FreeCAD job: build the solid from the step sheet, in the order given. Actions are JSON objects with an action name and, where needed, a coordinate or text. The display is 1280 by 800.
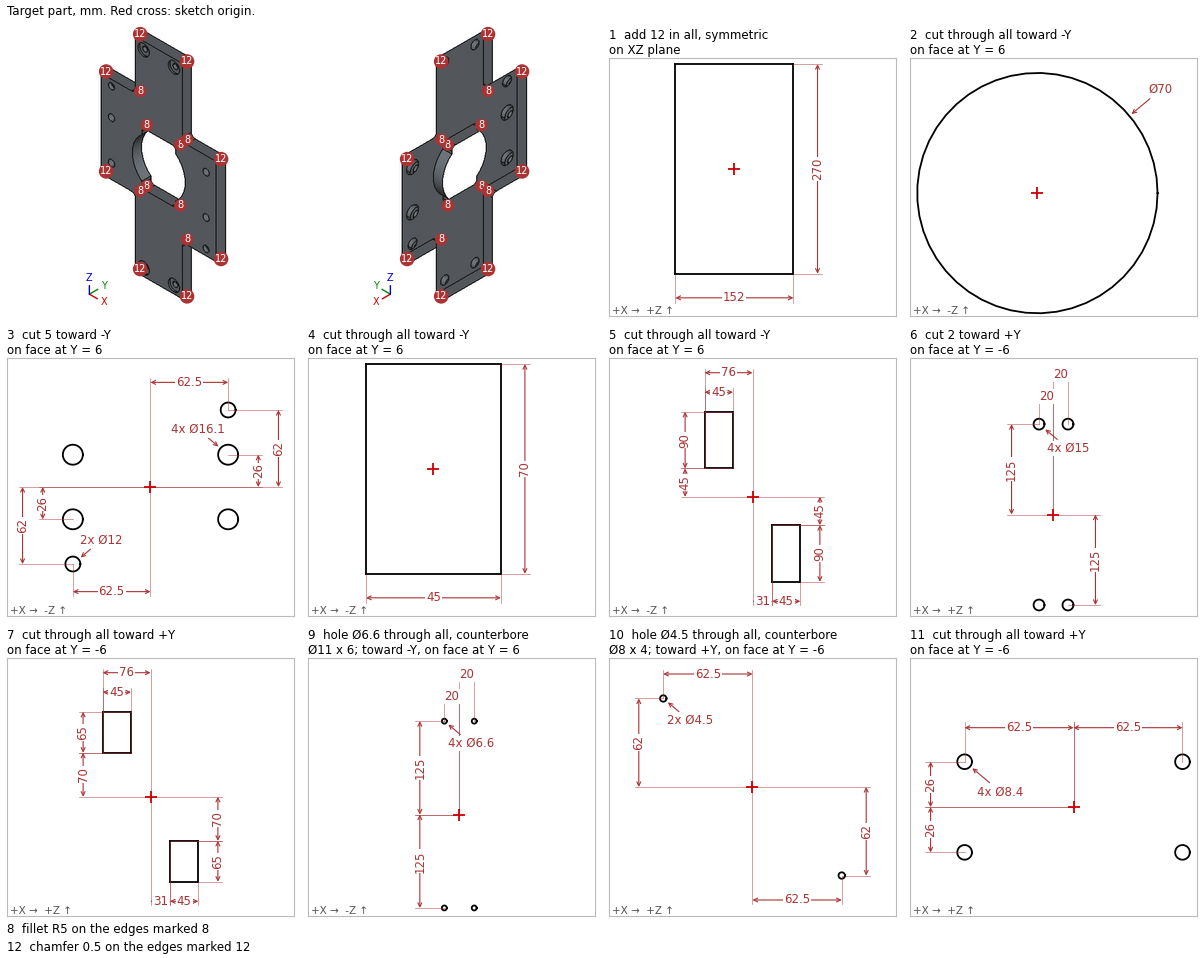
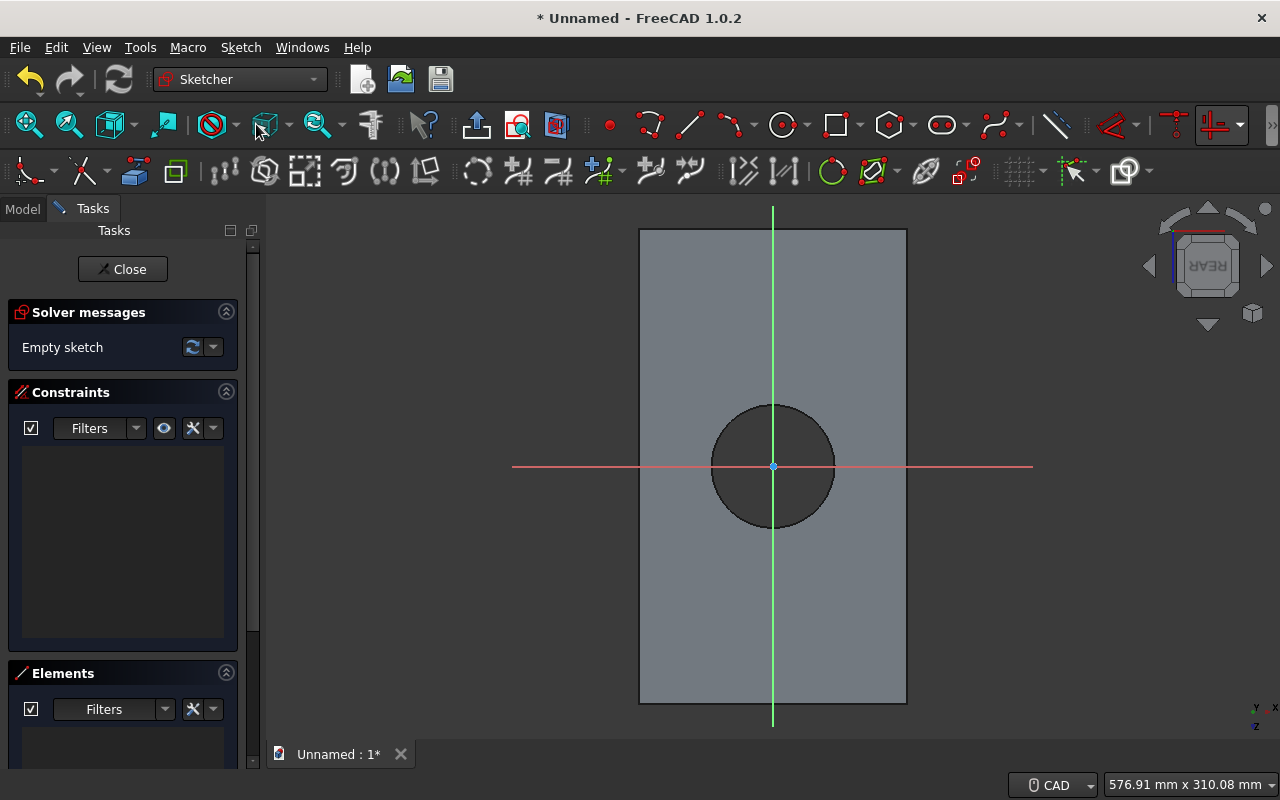
{"action": "scroll", "coordinate": [912, 466], "scroll_direction": "up", "scroll_amount": 2}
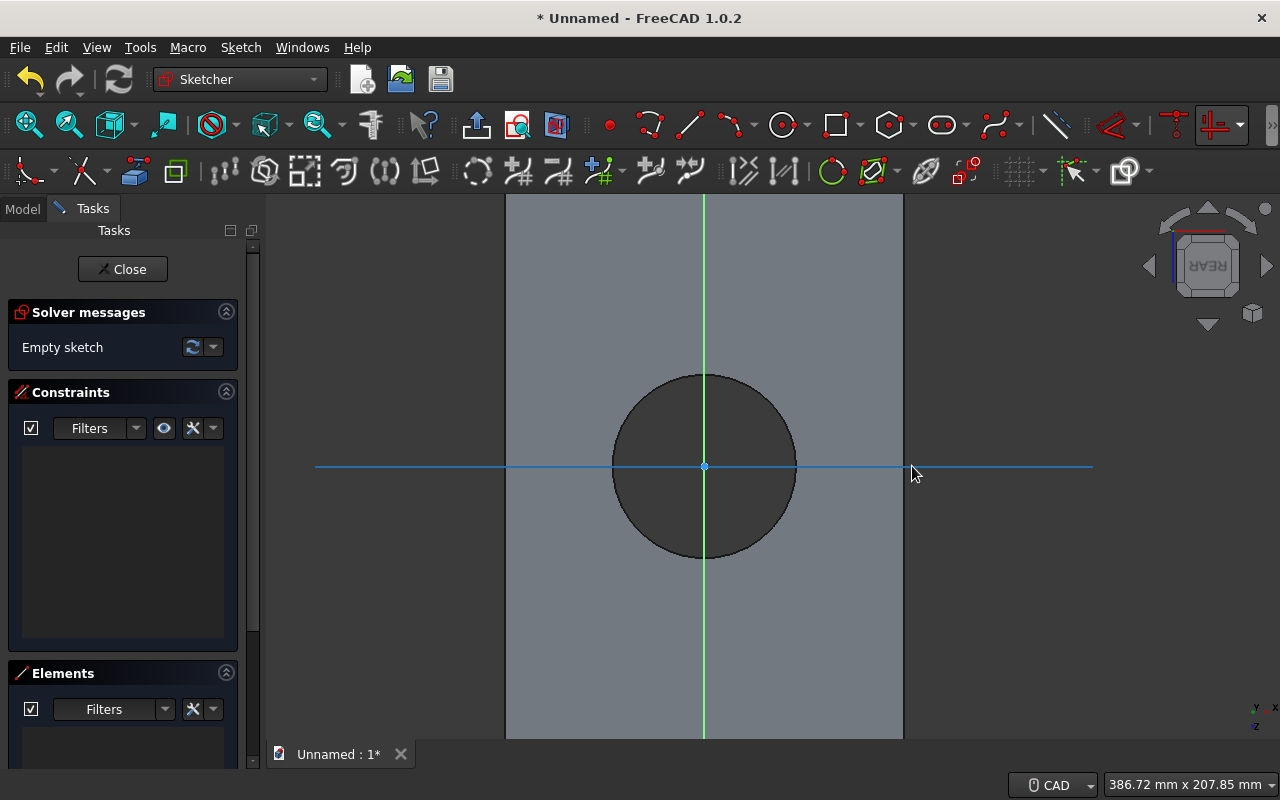
{"action": "left_click", "coordinate": [784, 126]}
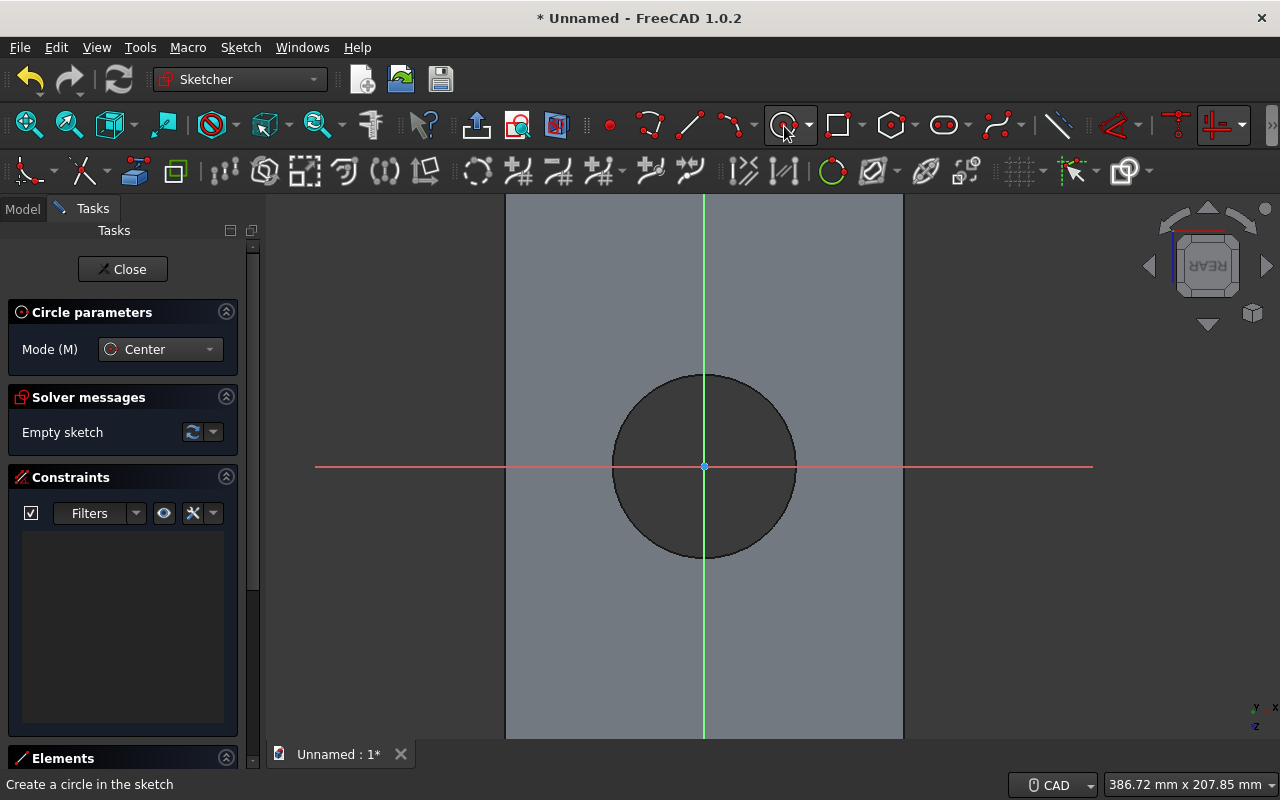
{"action": "scroll", "coordinate": [868, 304], "scroll_direction": "up", "scroll_amount": 2}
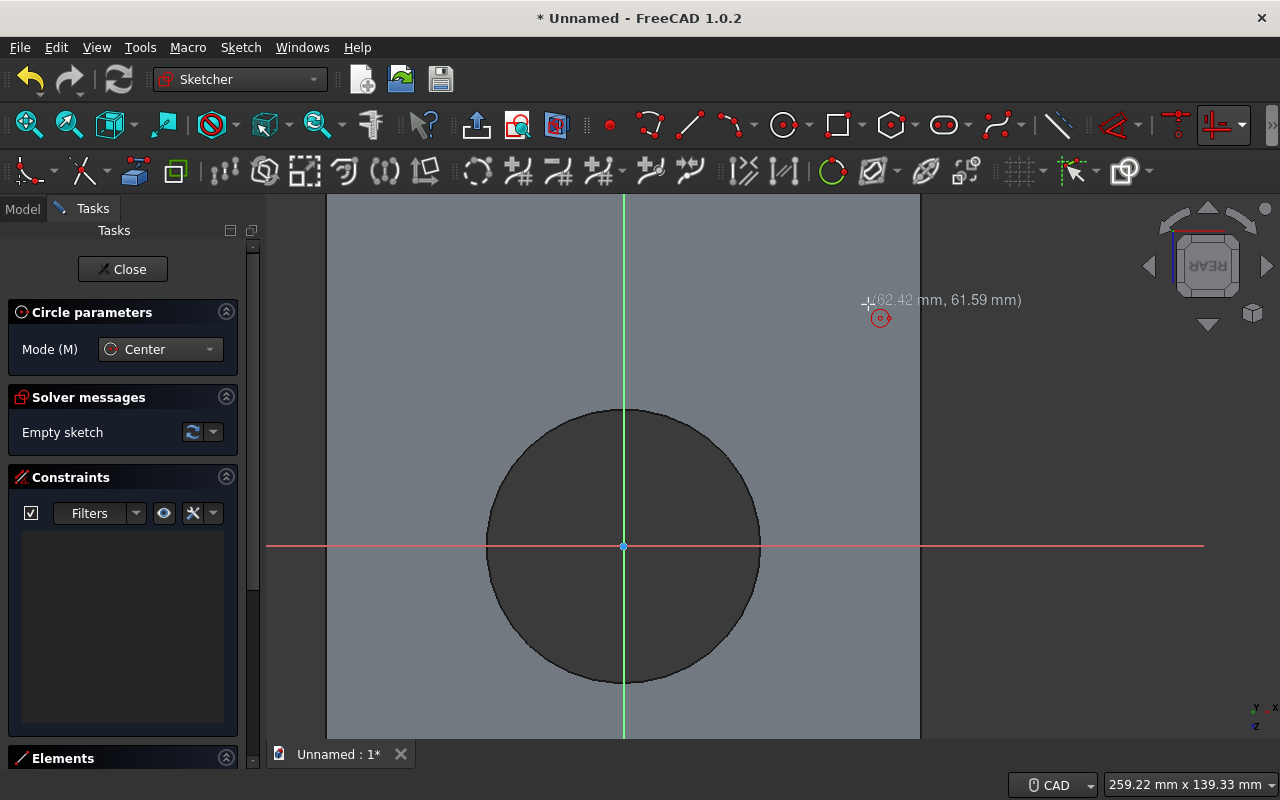
{"action": "left_click", "coordinate": [868, 304]}
{"action": "mouse_move", "coordinate": [885, 287]}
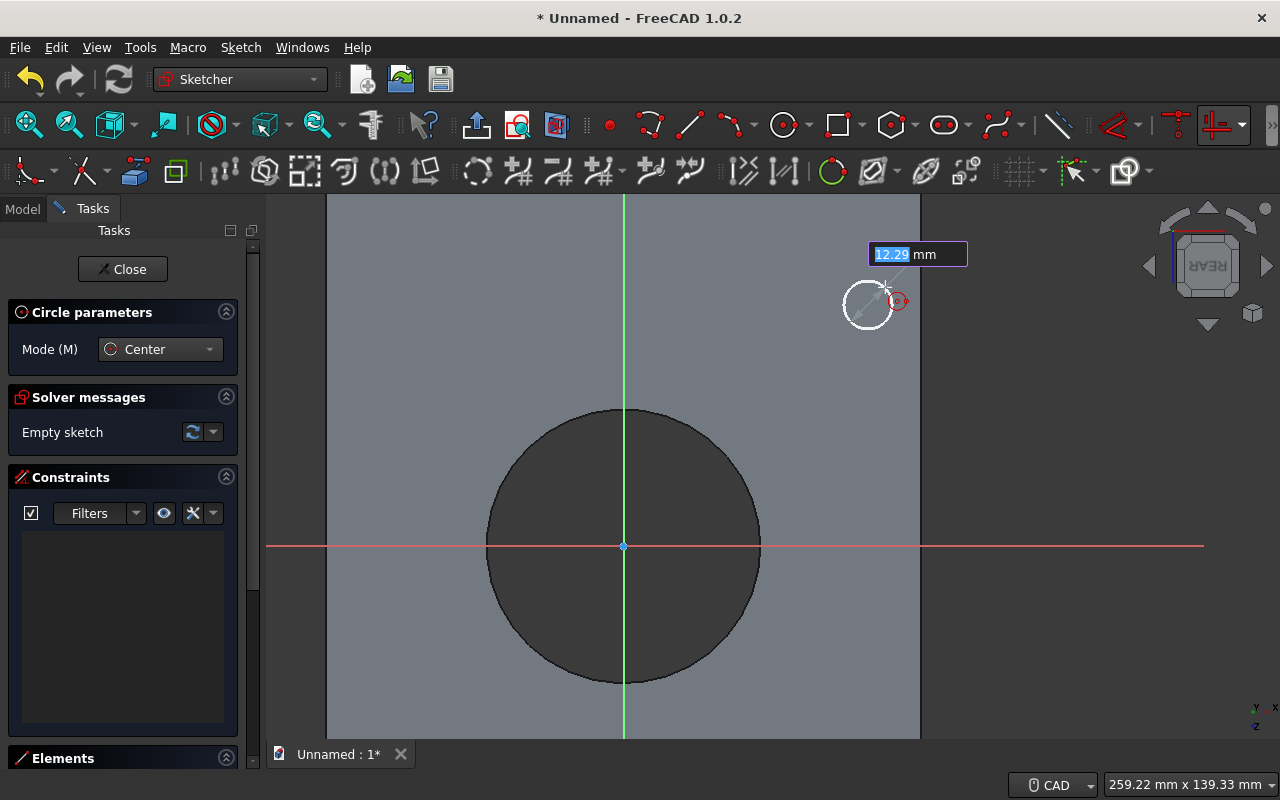
{"action": "type", "text": "12"}
{"action": "key", "text": "Return"}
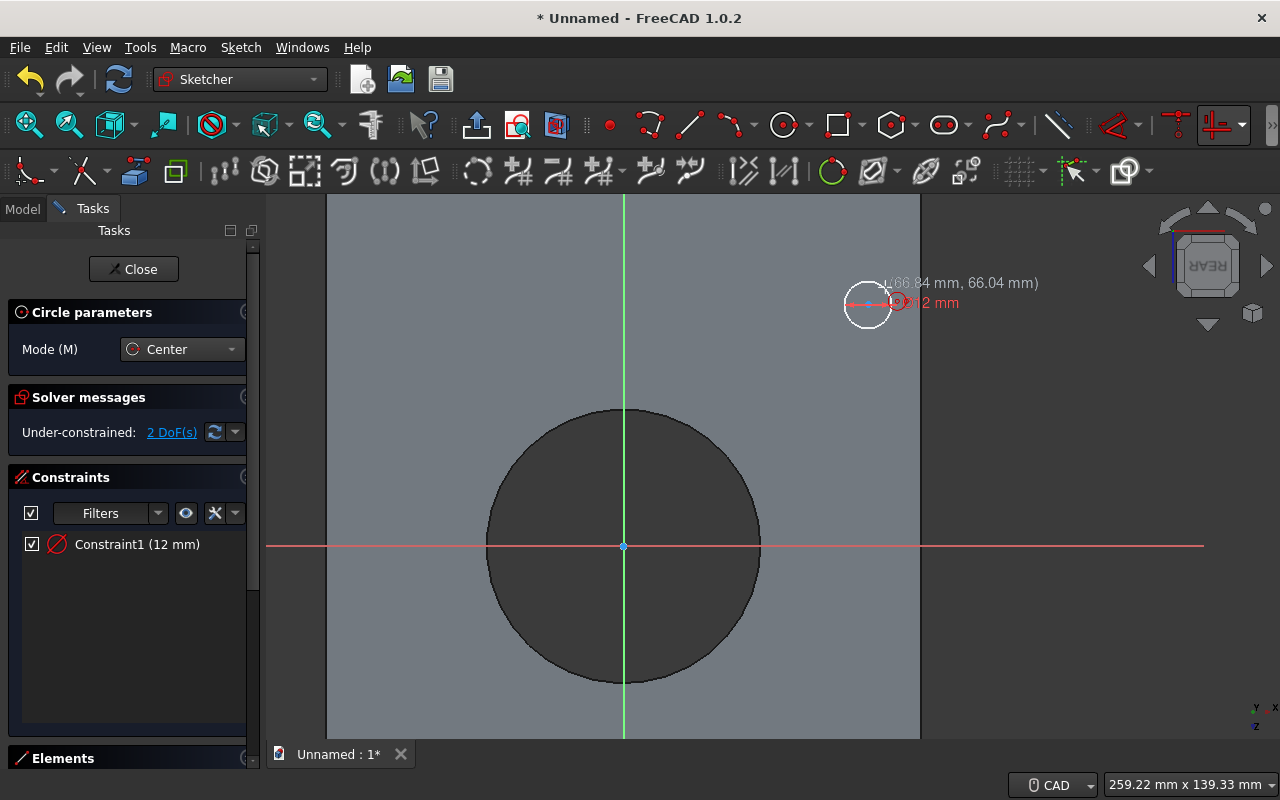
{"action": "scroll", "coordinate": [869, 304], "scroll_direction": "down", "scroll_amount": 2}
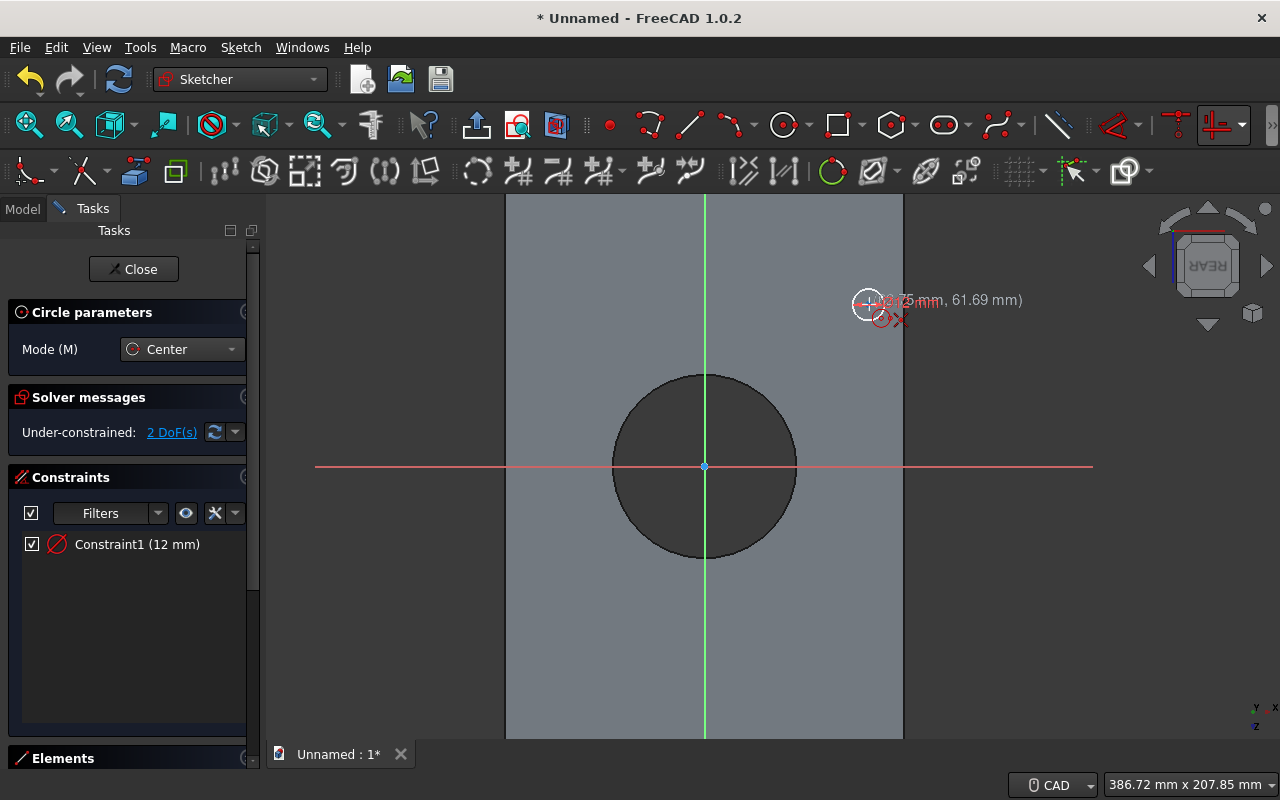
{"action": "scroll", "coordinate": [541, 629], "scroll_direction": "up", "scroll_amount": 2}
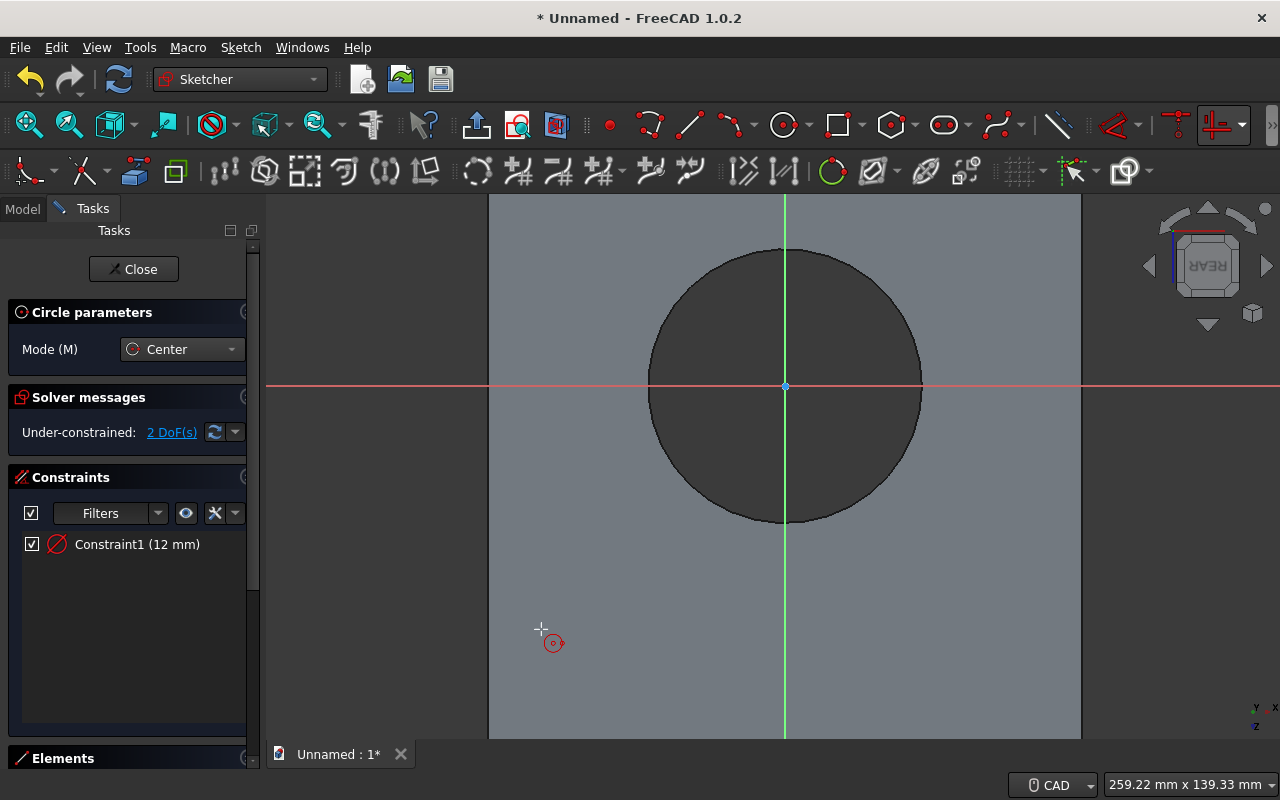
{"action": "left_click", "coordinate": [541, 629]}
{"action": "mouse_move", "coordinate": [557, 612]}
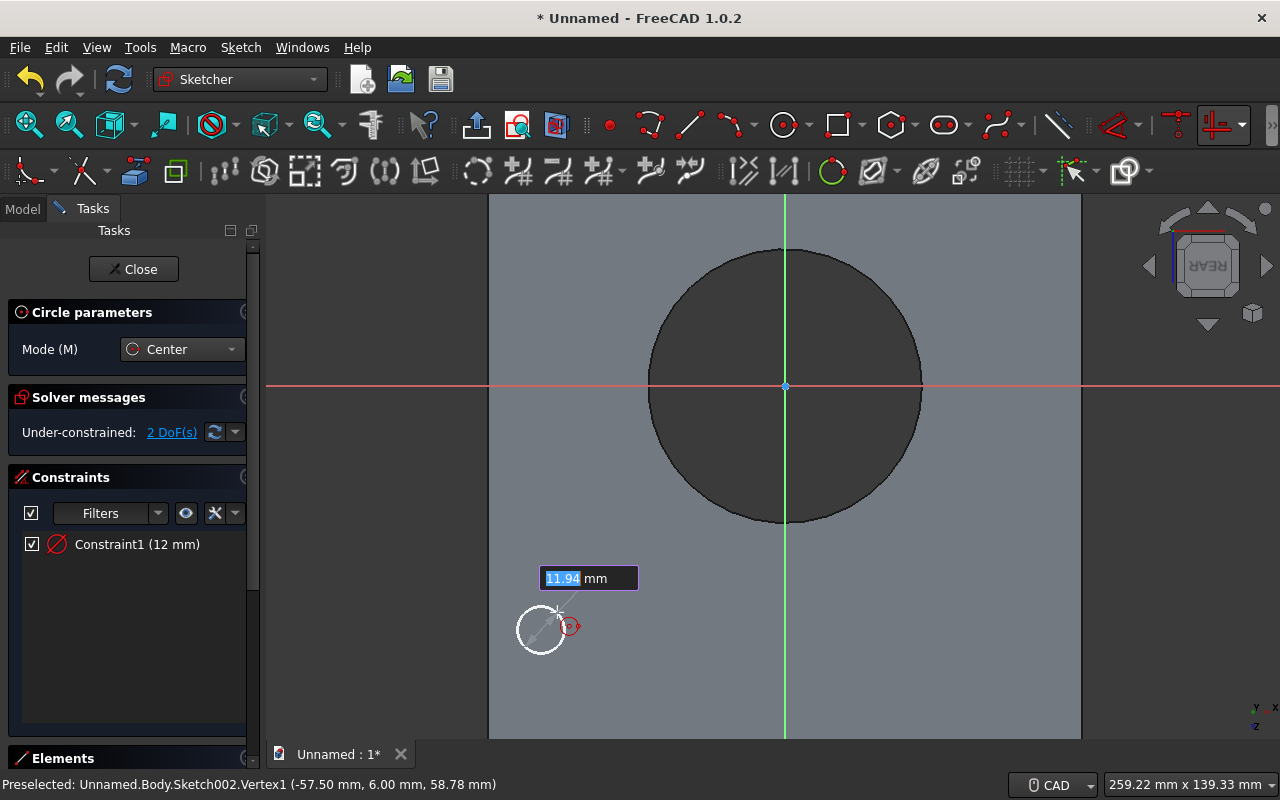
{"action": "type", "text": "12"}
{"action": "key", "text": "Return"}